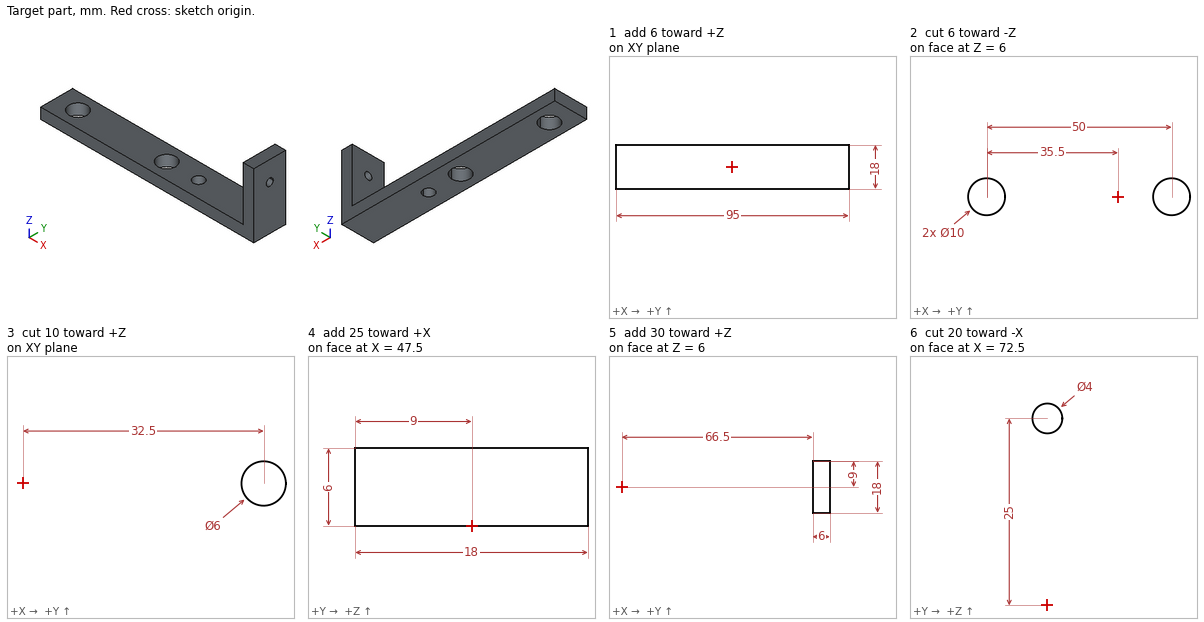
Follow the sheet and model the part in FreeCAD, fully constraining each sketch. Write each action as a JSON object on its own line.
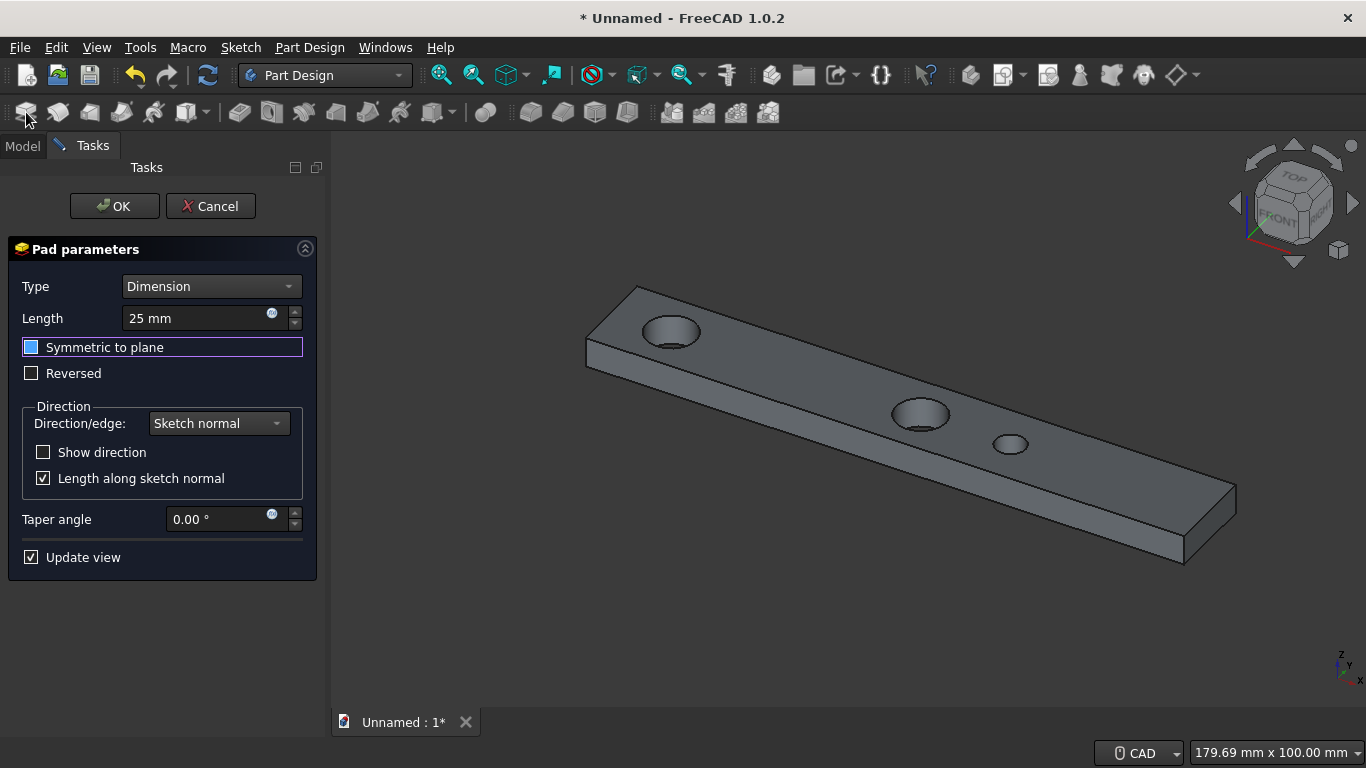
{"action": "left_click", "coordinate": [115, 206]}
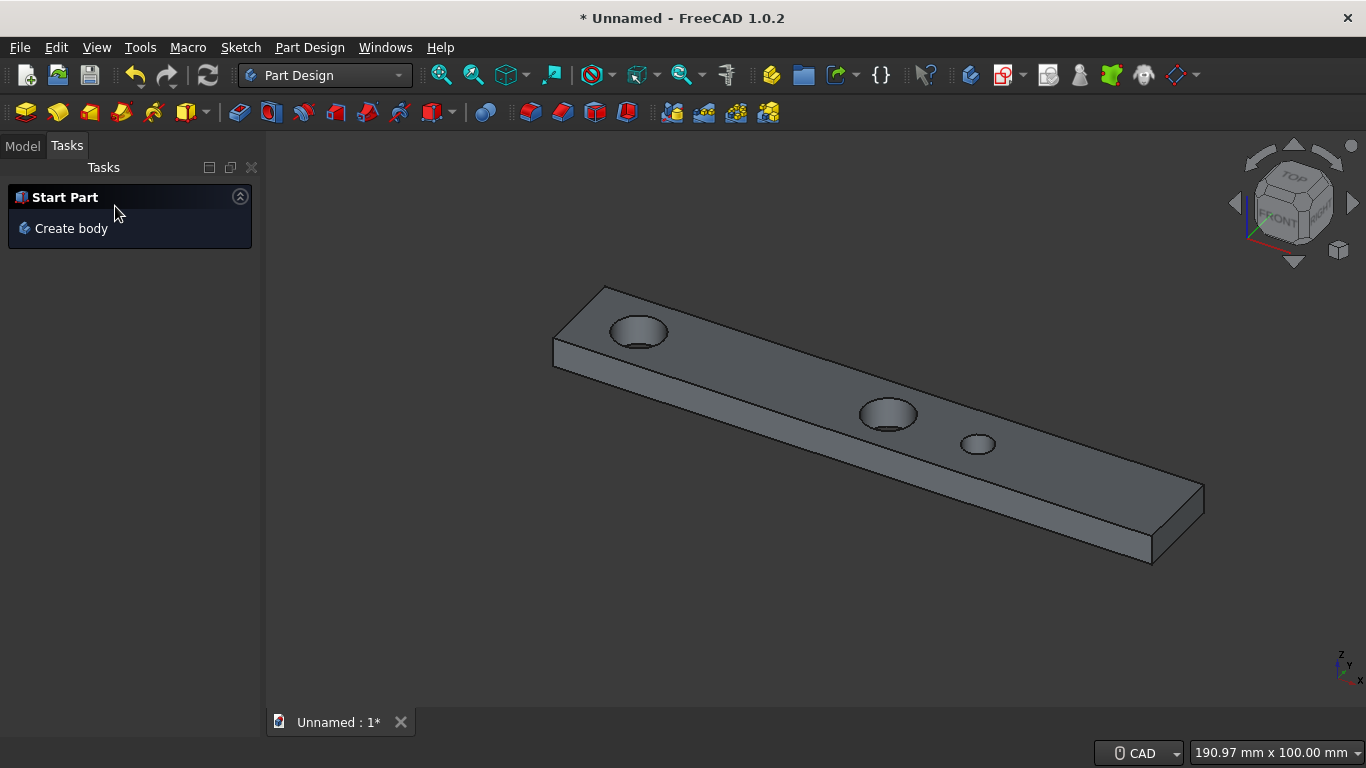
{"action": "left_click", "coordinate": [1049, 467]}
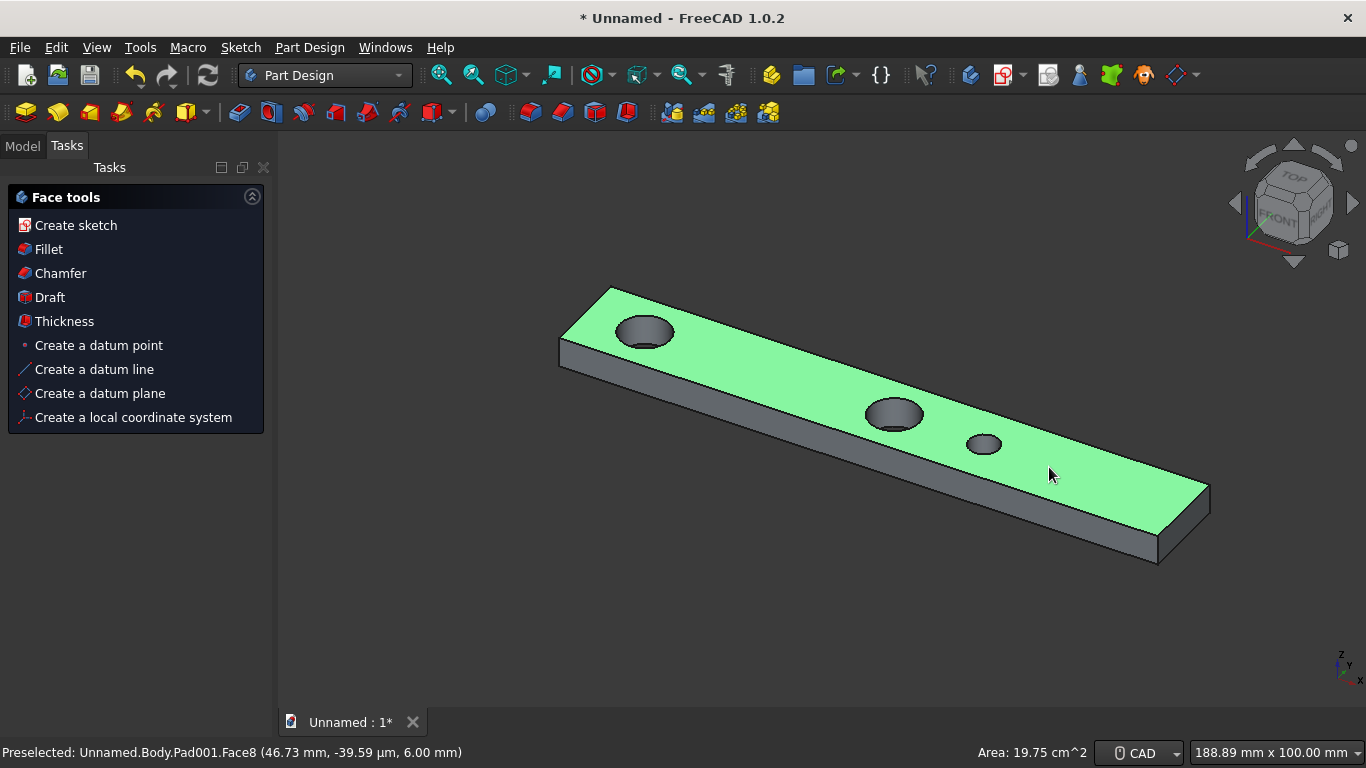
{"action": "left_click", "coordinate": [1004, 76]}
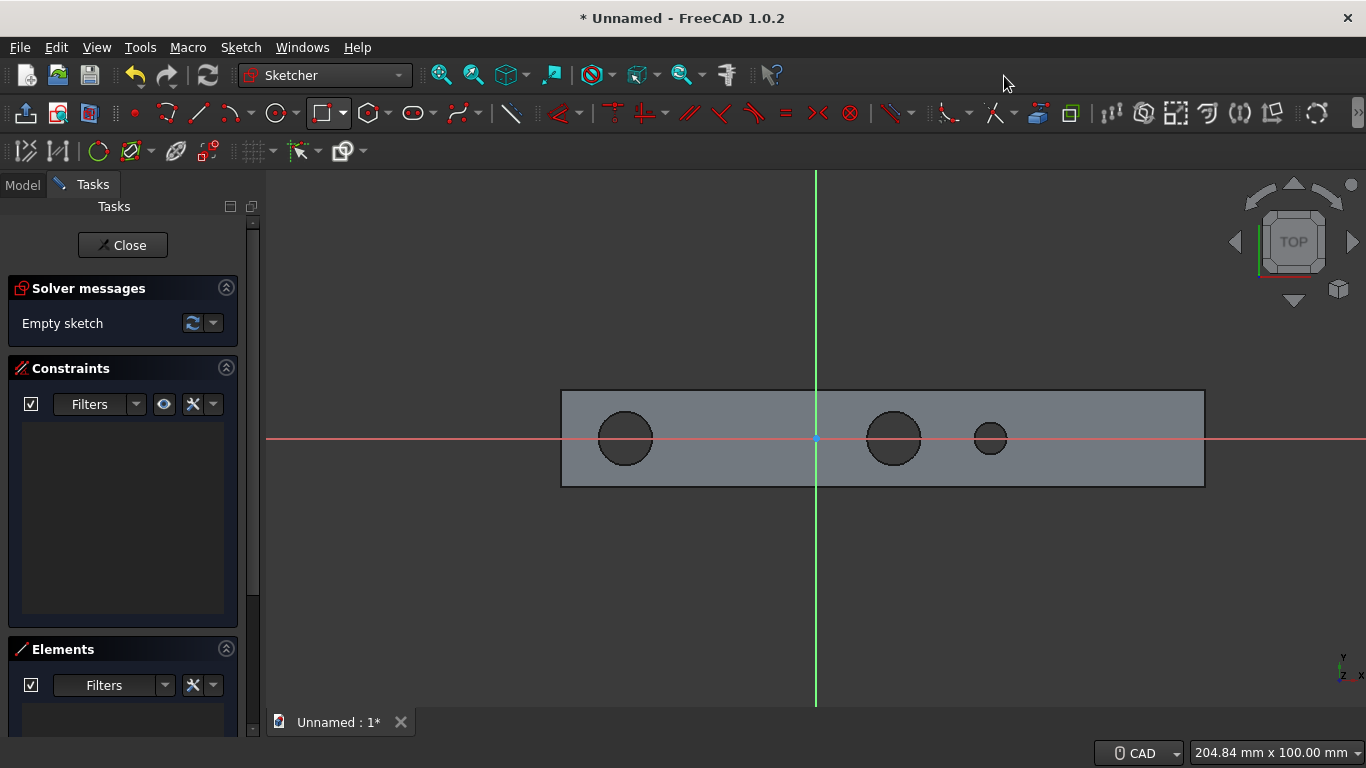
{"action": "scroll", "coordinate": [748, 438], "scroll_direction": "down", "scroll_amount": 5}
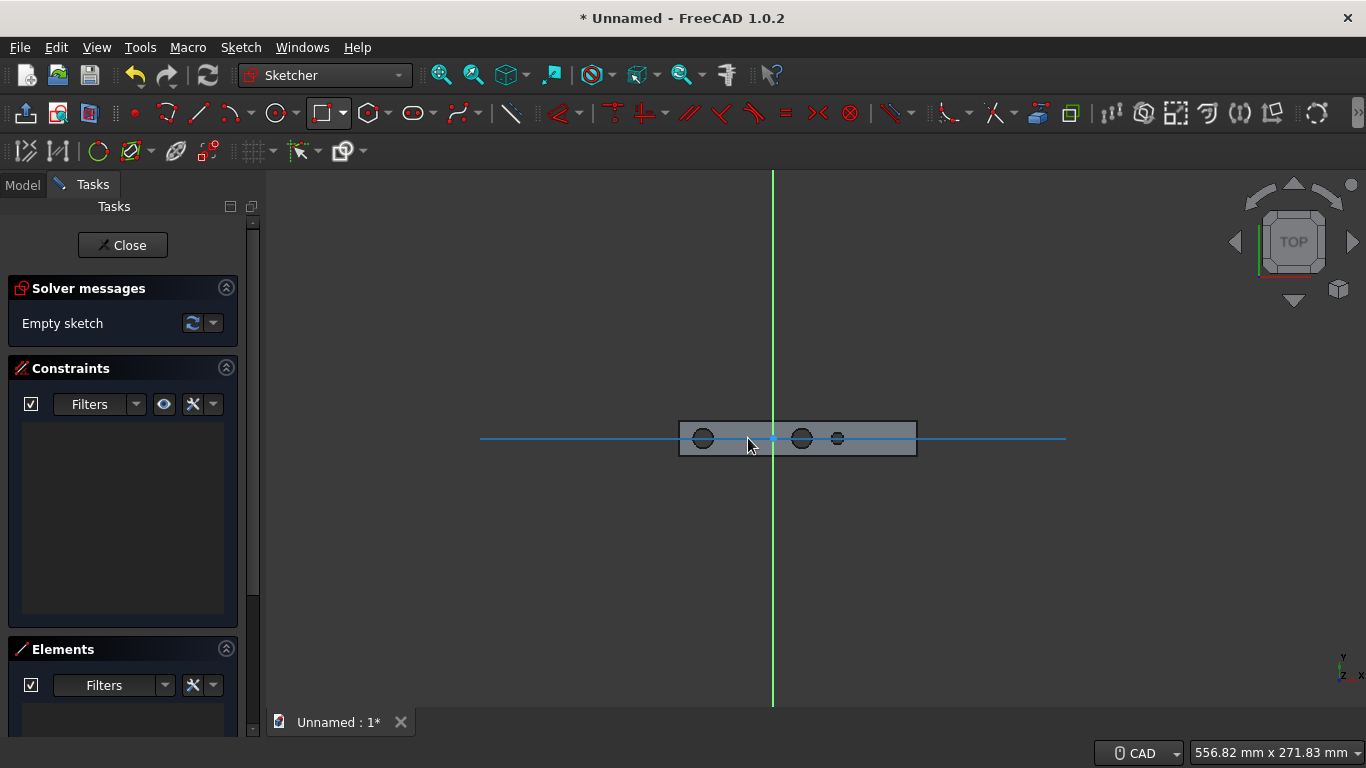
{"action": "scroll", "coordinate": [931, 438], "scroll_direction": "up", "scroll_amount": 11}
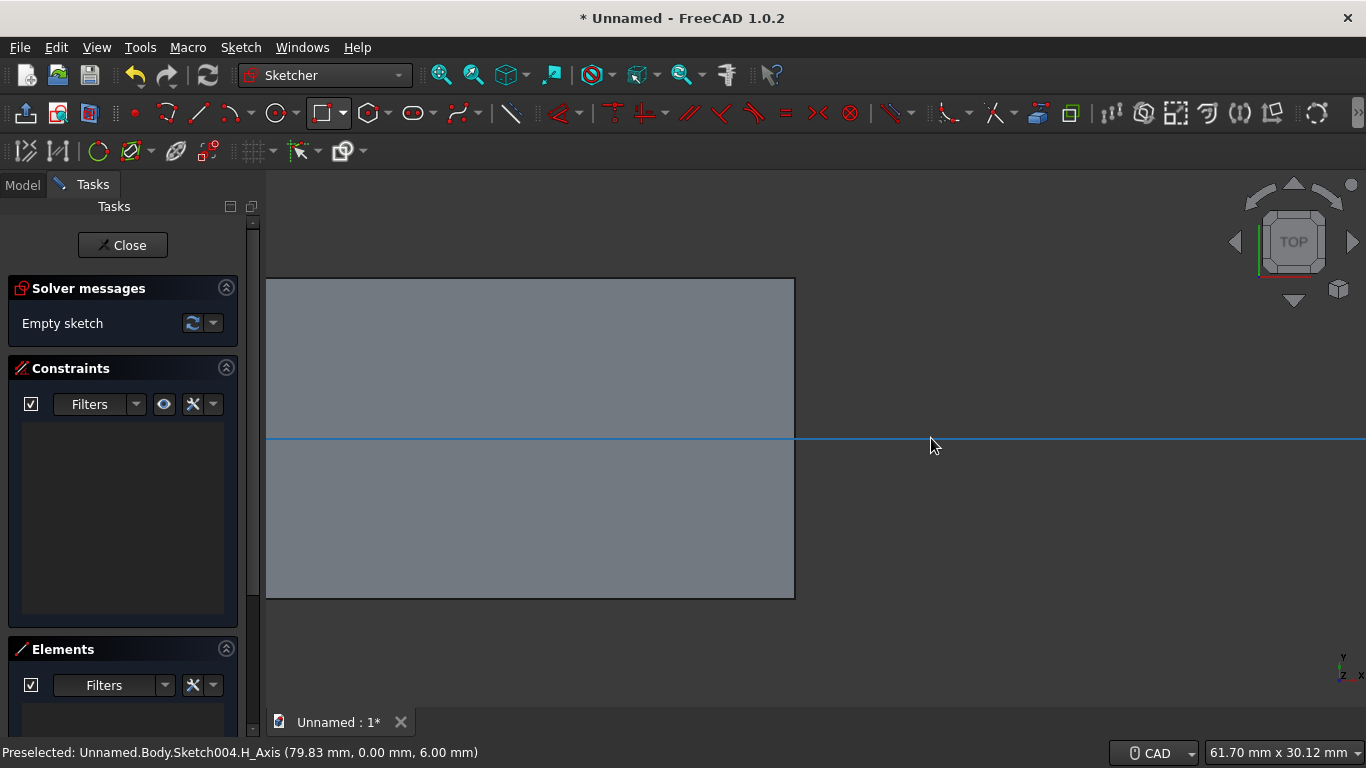
{"action": "left_click", "coordinate": [322, 114]}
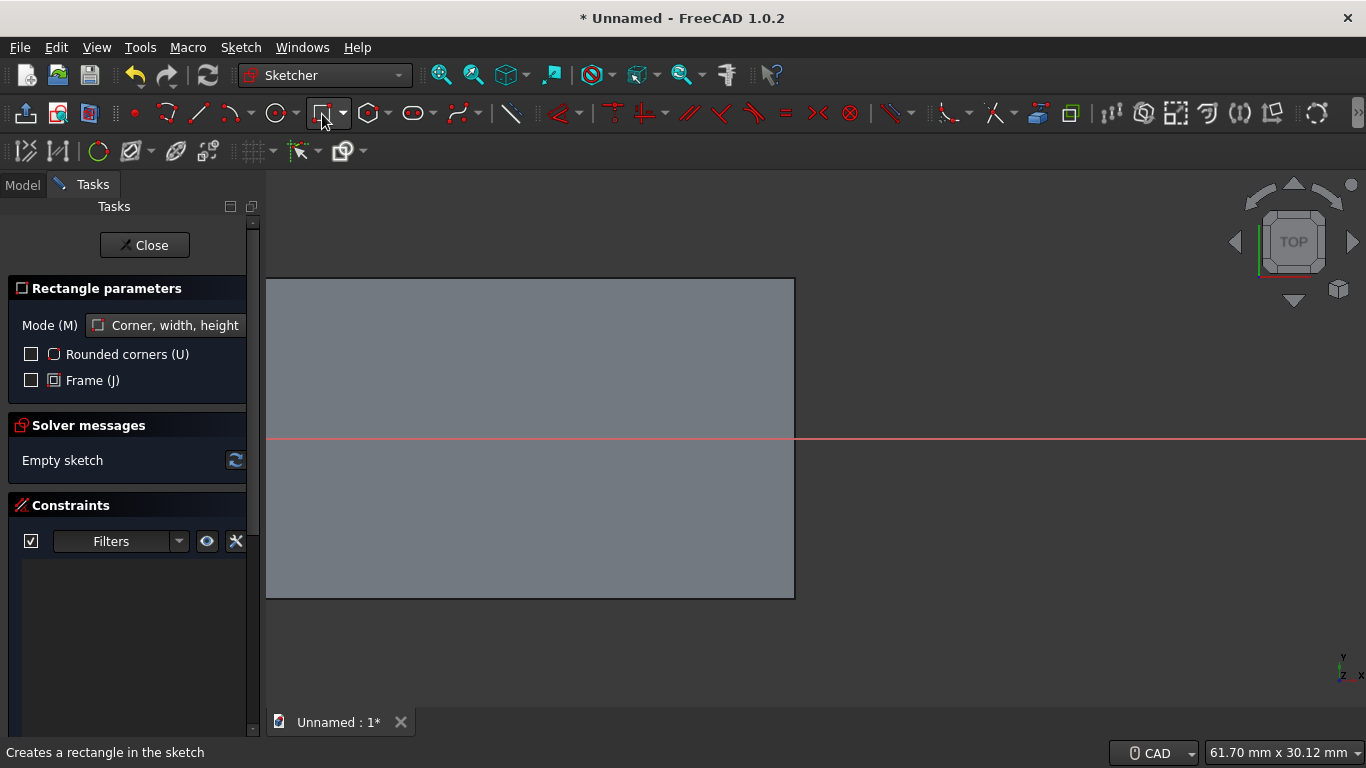
{"action": "left_click", "coordinate": [688, 278]}
{"action": "left_click", "coordinate": [795, 599]}
{"action": "key", "text": "Escape"}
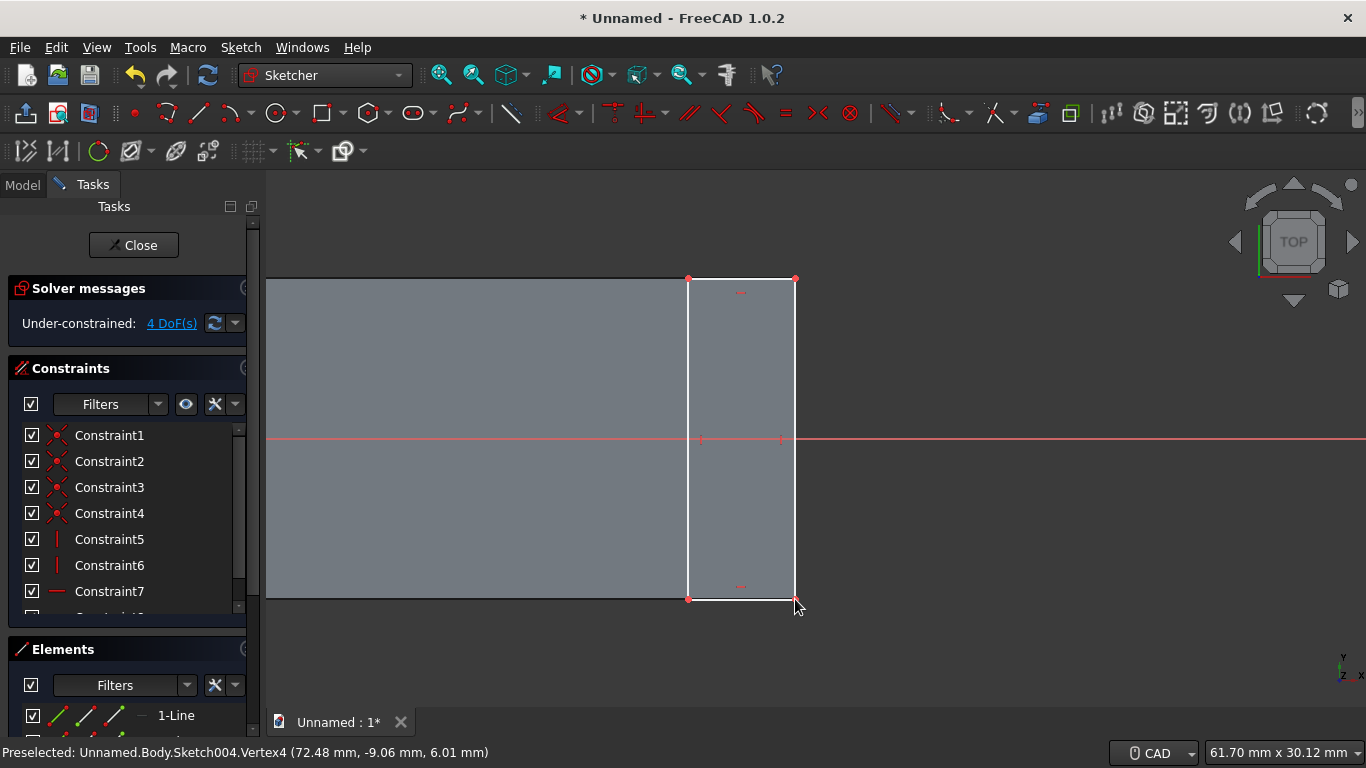
{"action": "left_click", "coordinate": [558, 114]}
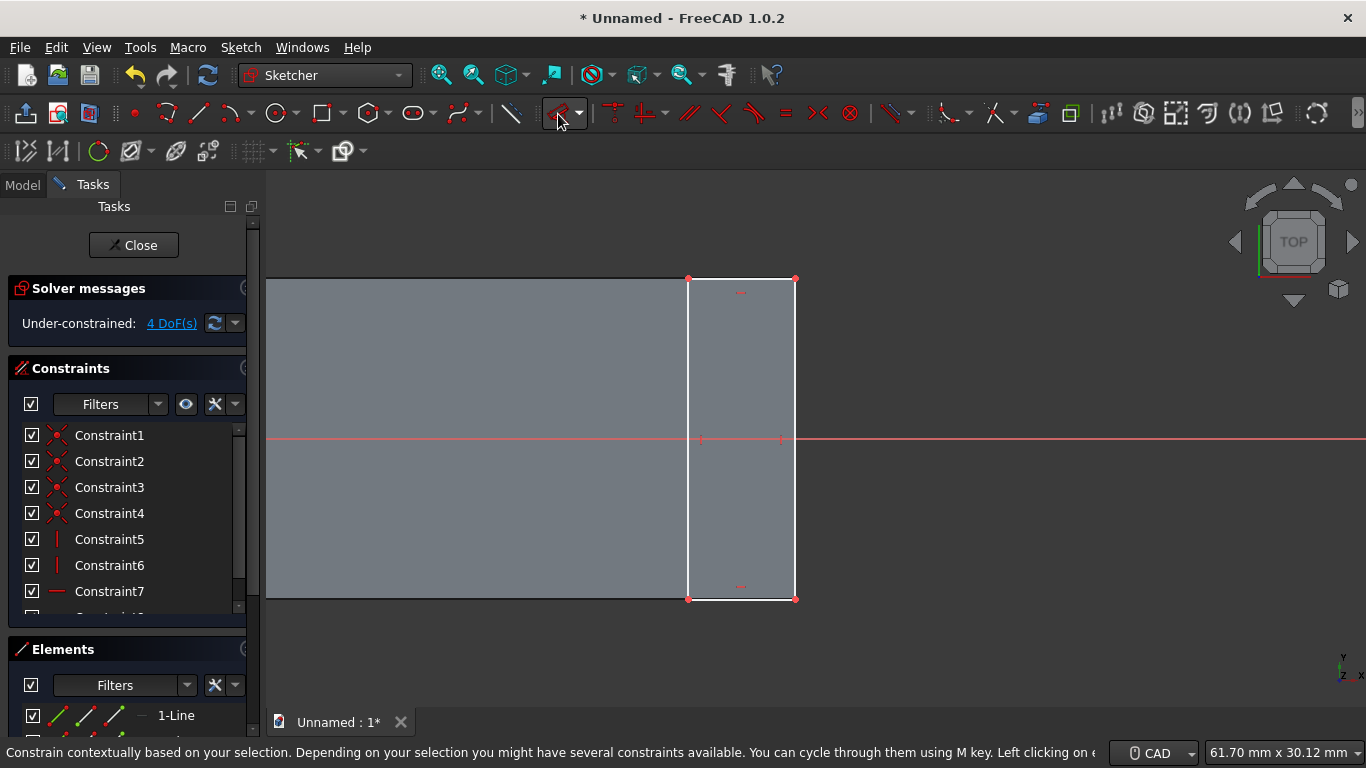
{"action": "left_click", "coordinate": [720, 600]}
{"action": "left_click", "coordinate": [741, 634]}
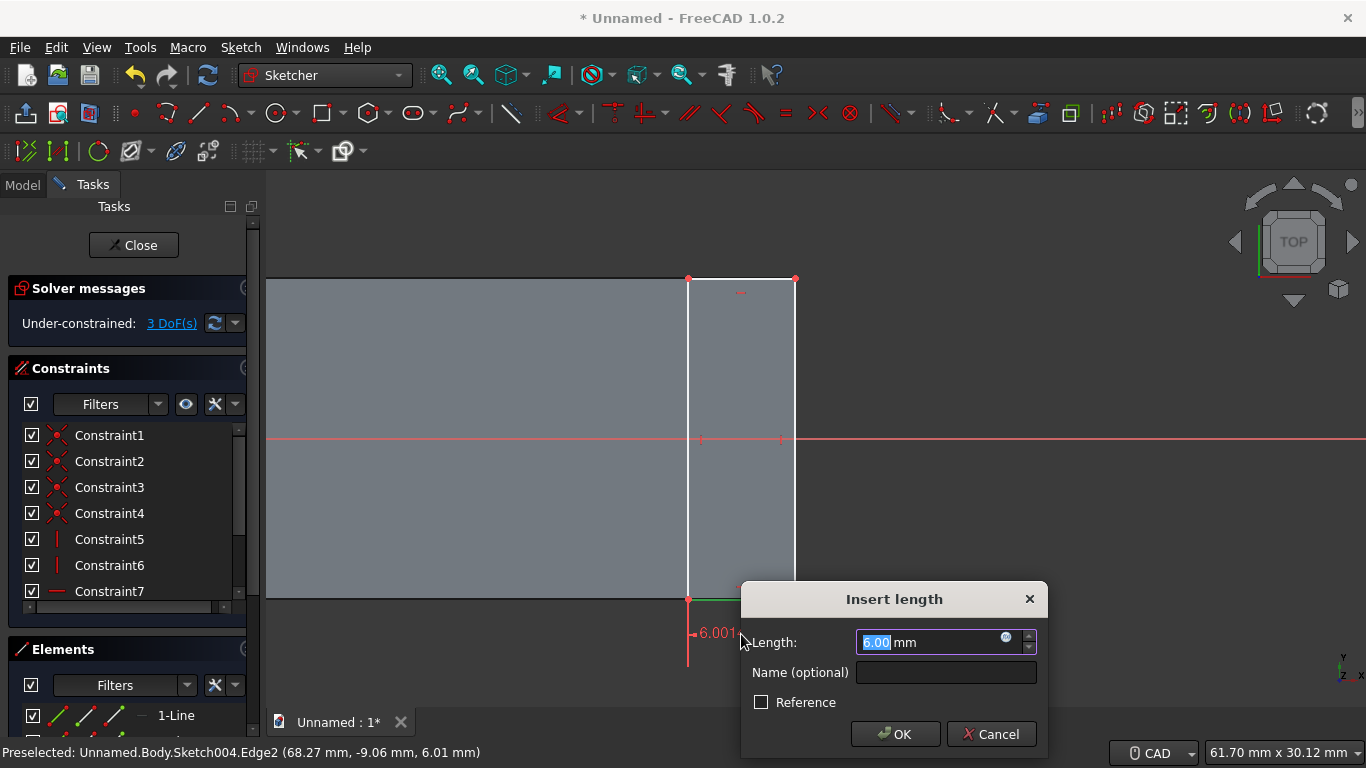
{"action": "type", "text": "6"}
{"action": "key", "text": "Return"}